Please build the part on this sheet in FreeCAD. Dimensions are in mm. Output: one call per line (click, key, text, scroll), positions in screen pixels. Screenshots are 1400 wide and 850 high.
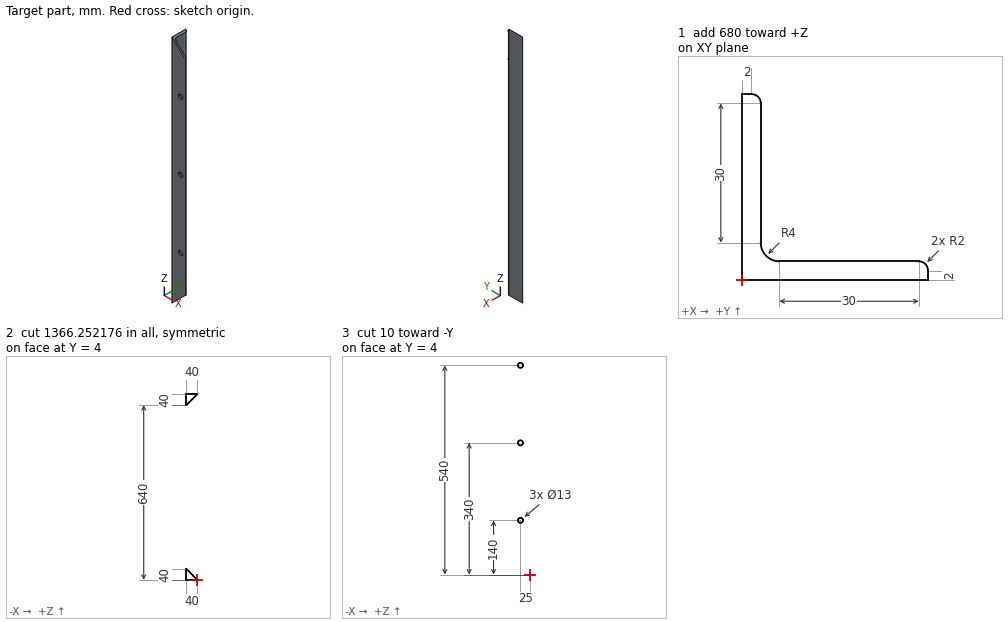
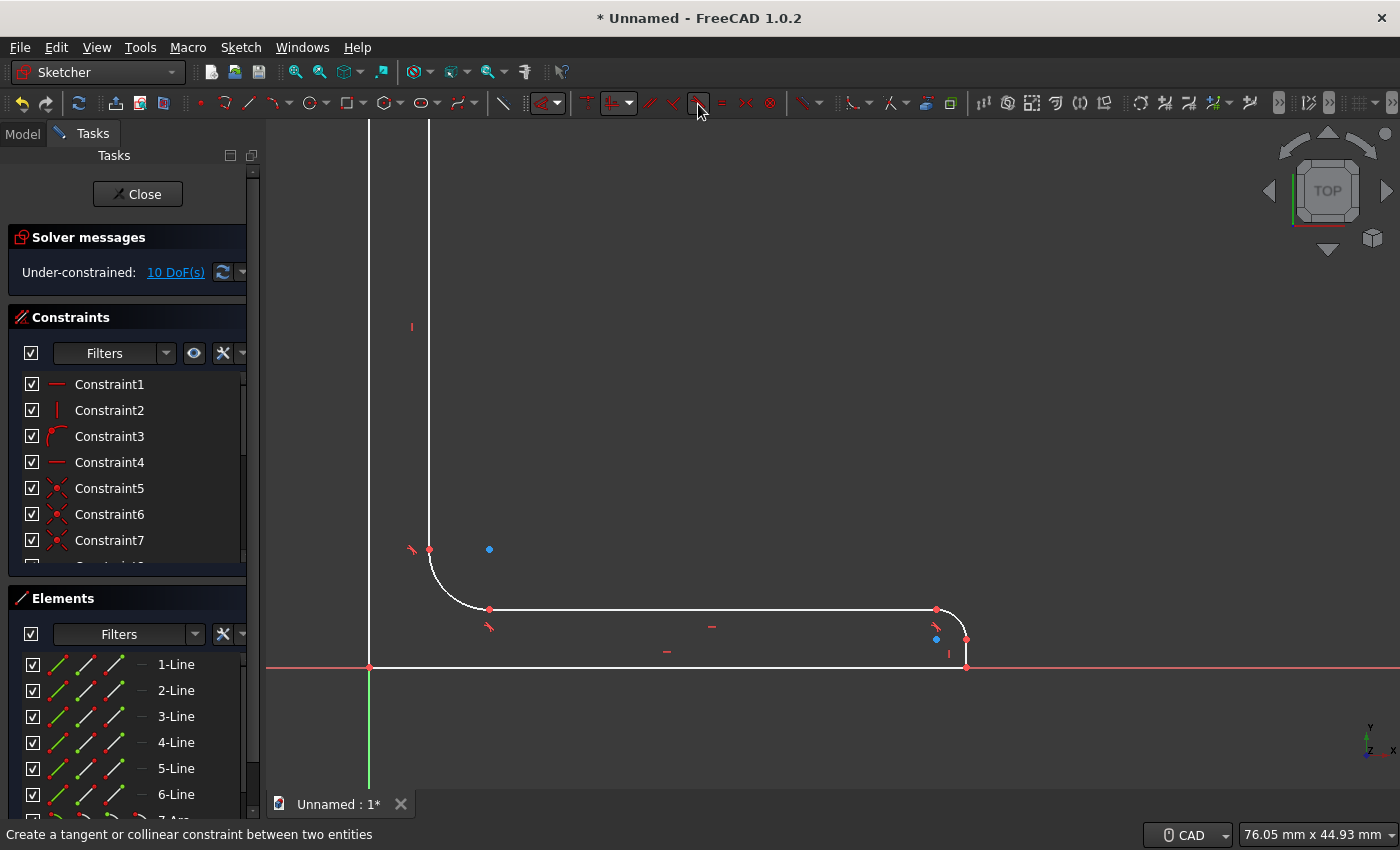
click(429, 416)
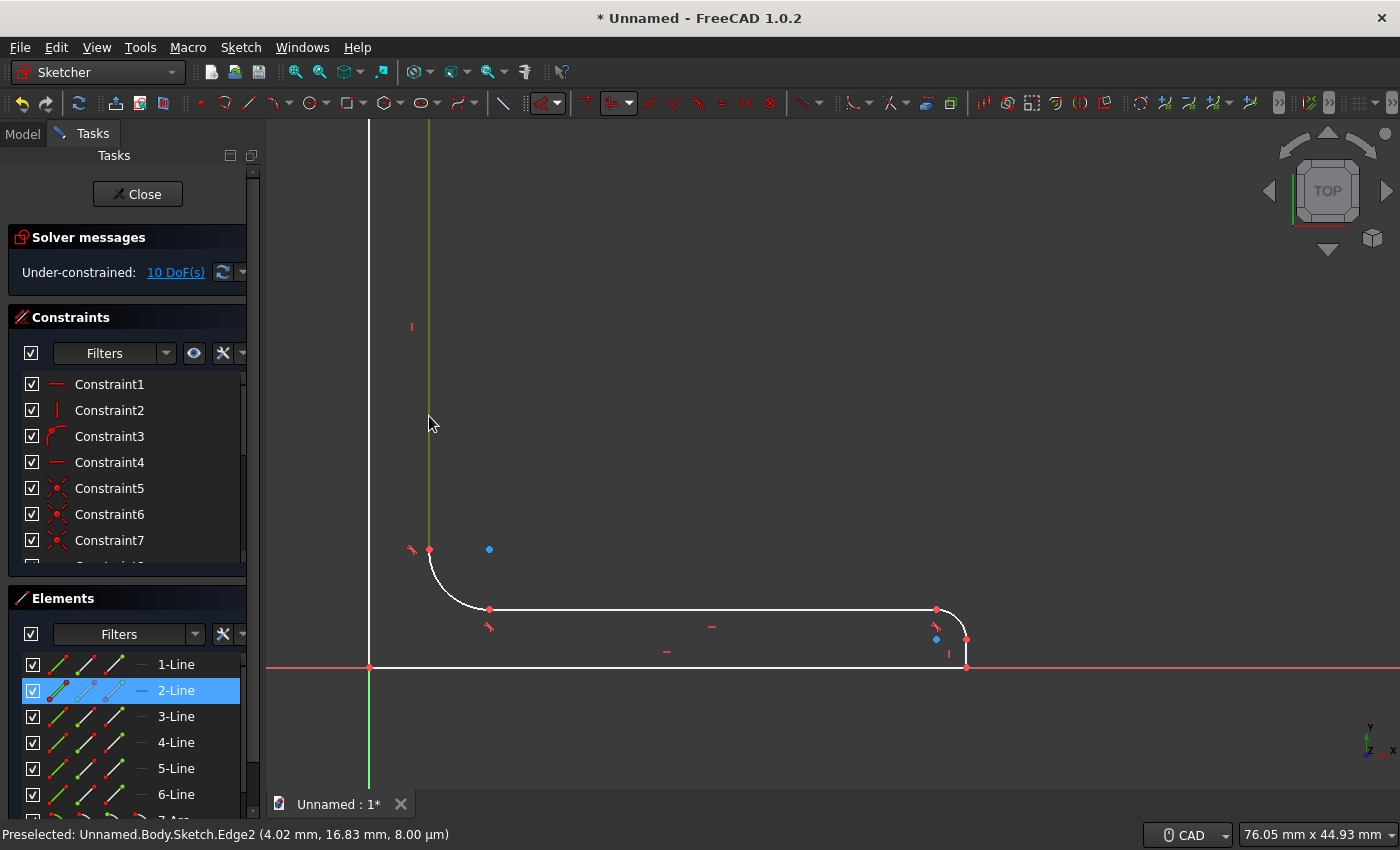
scroll(962, 625, down, 2)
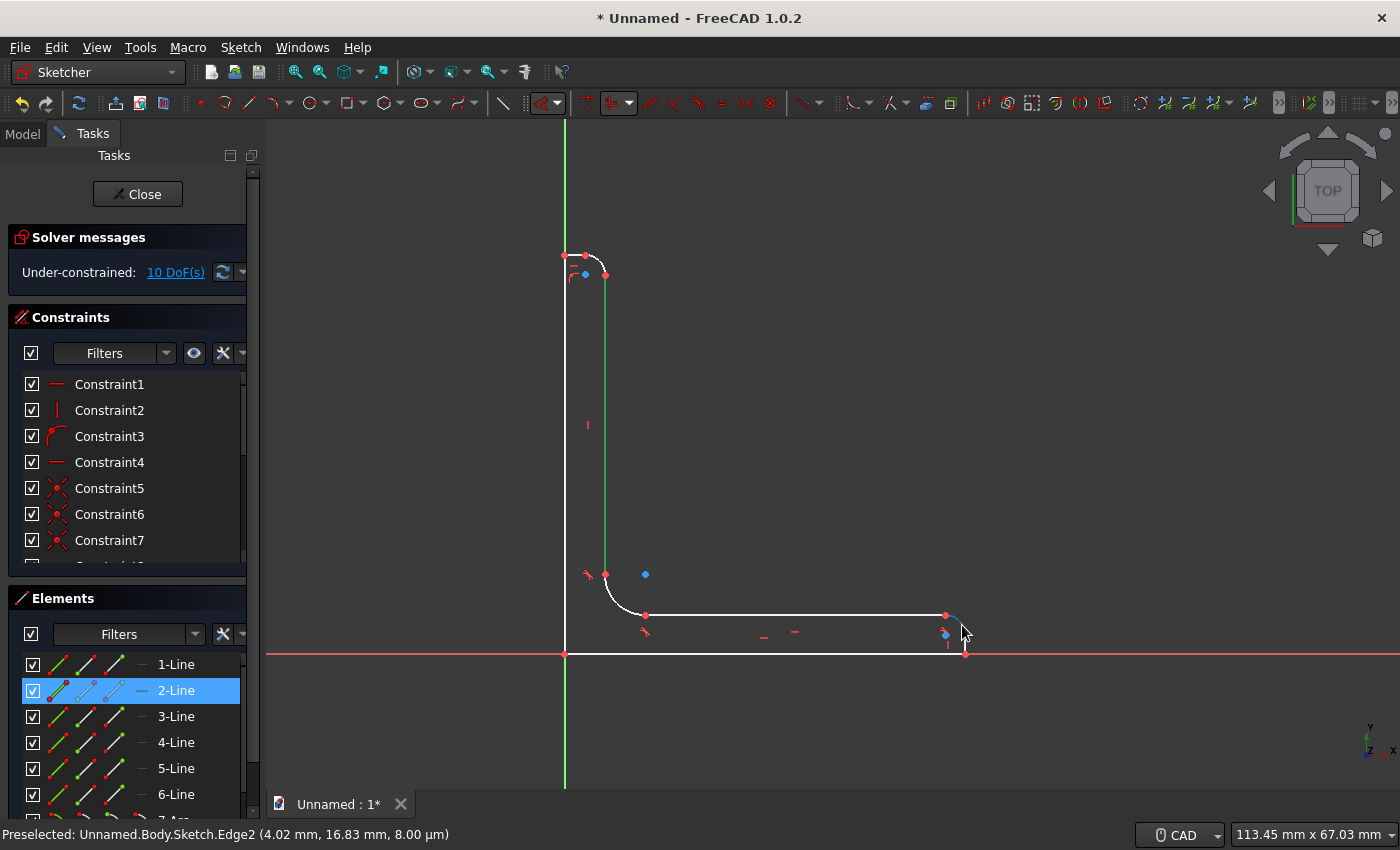
scroll(603, 266, up, 2)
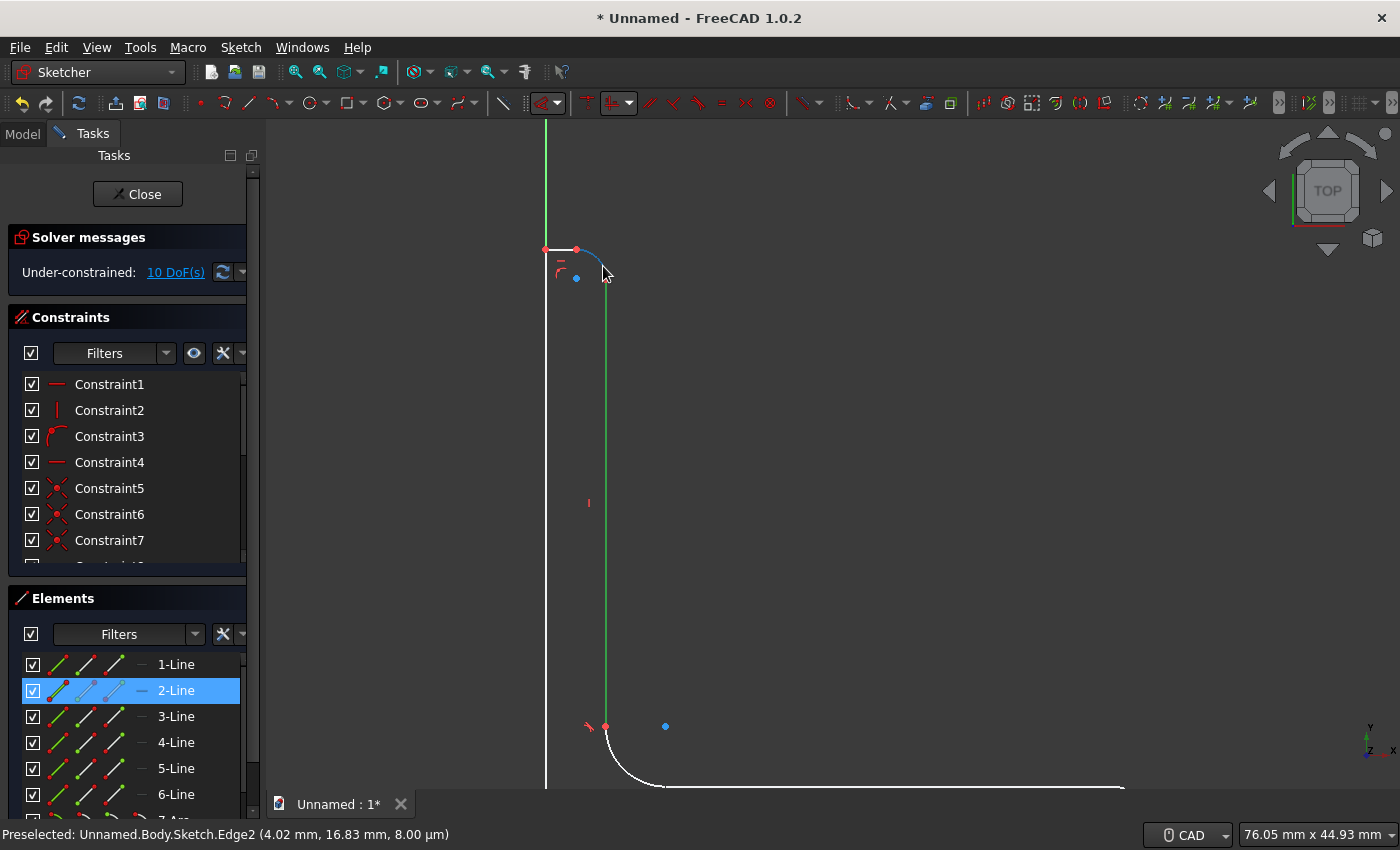
click(603, 266)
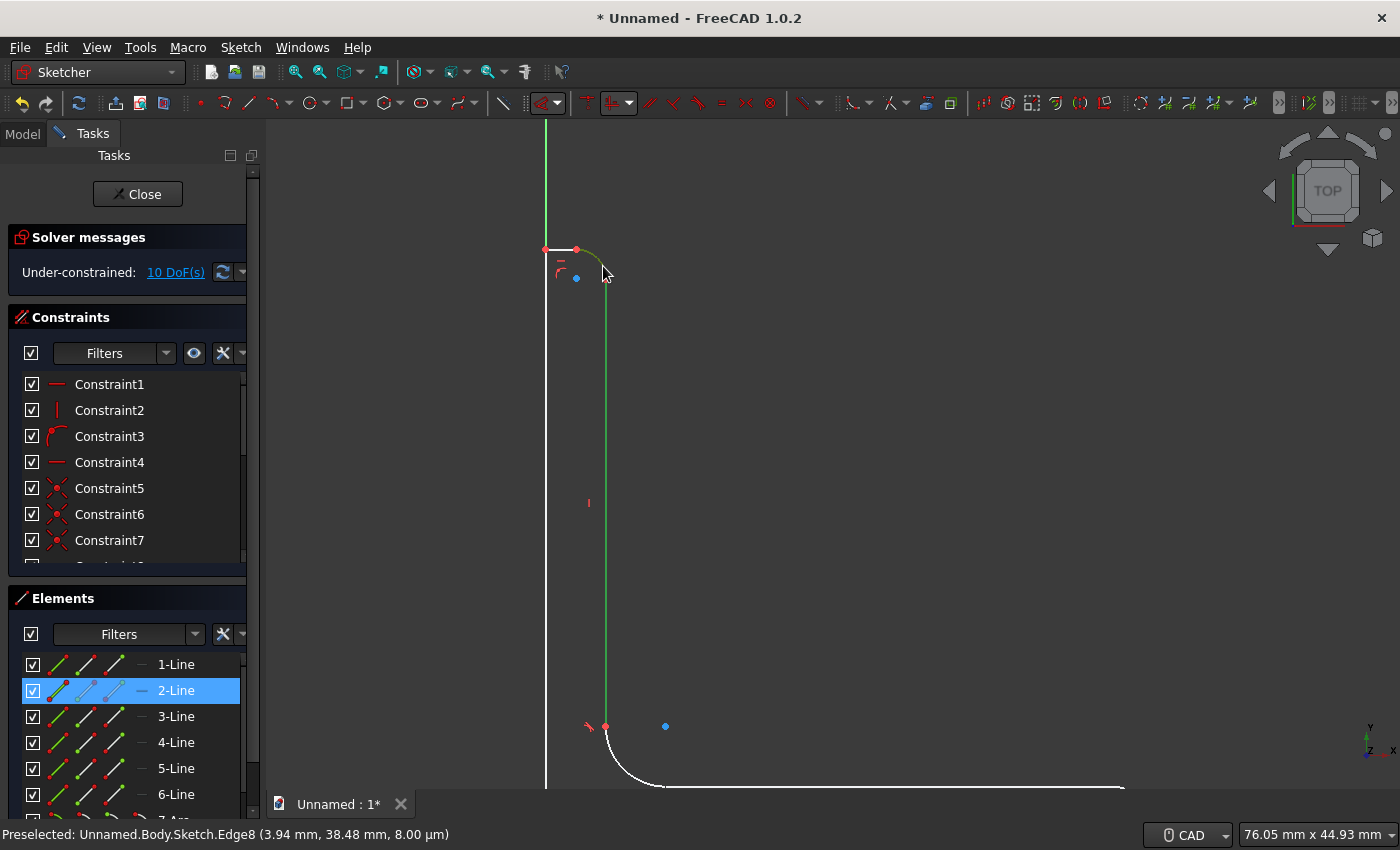
click(698, 104)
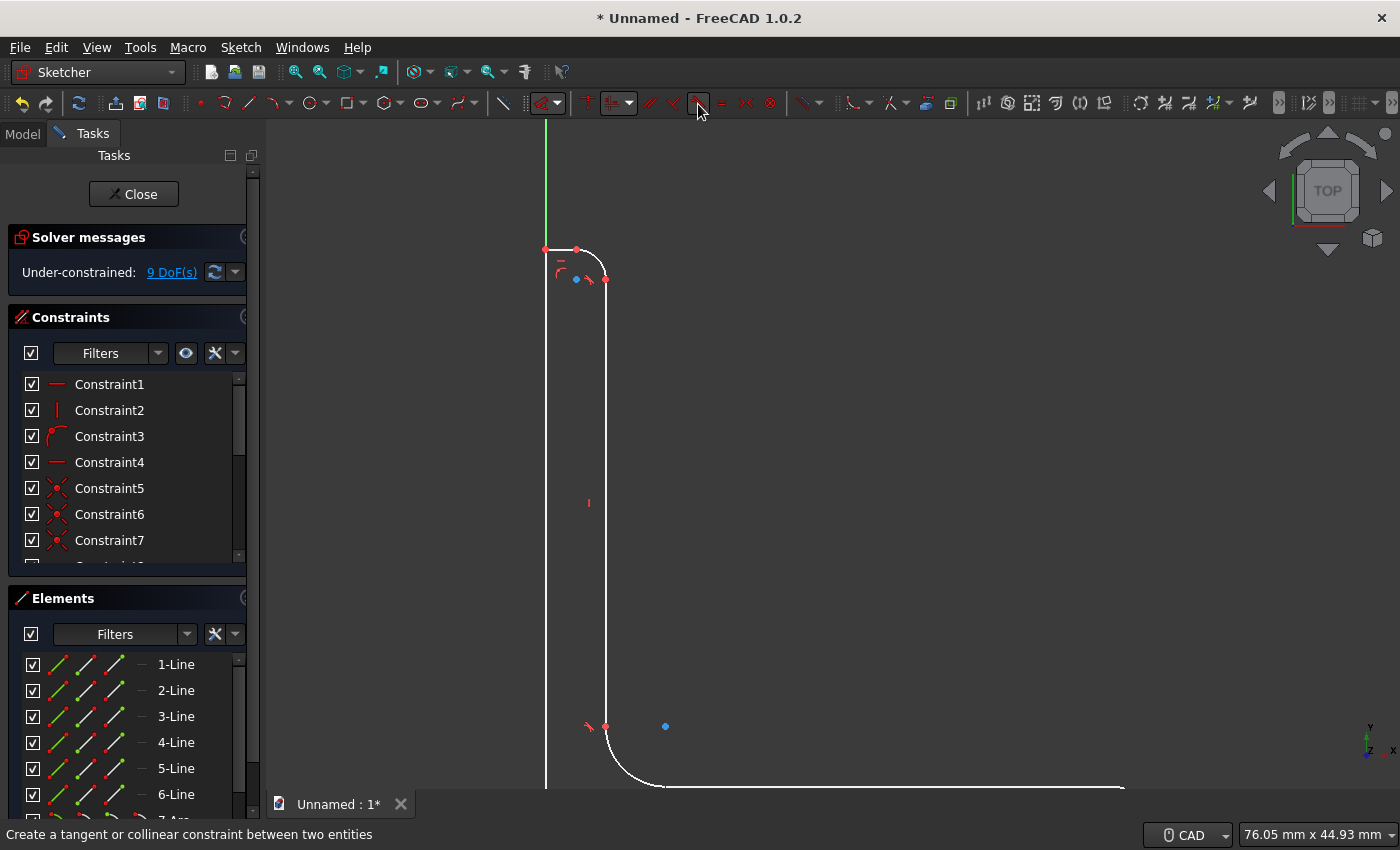
scroll(567, 250, up, 3)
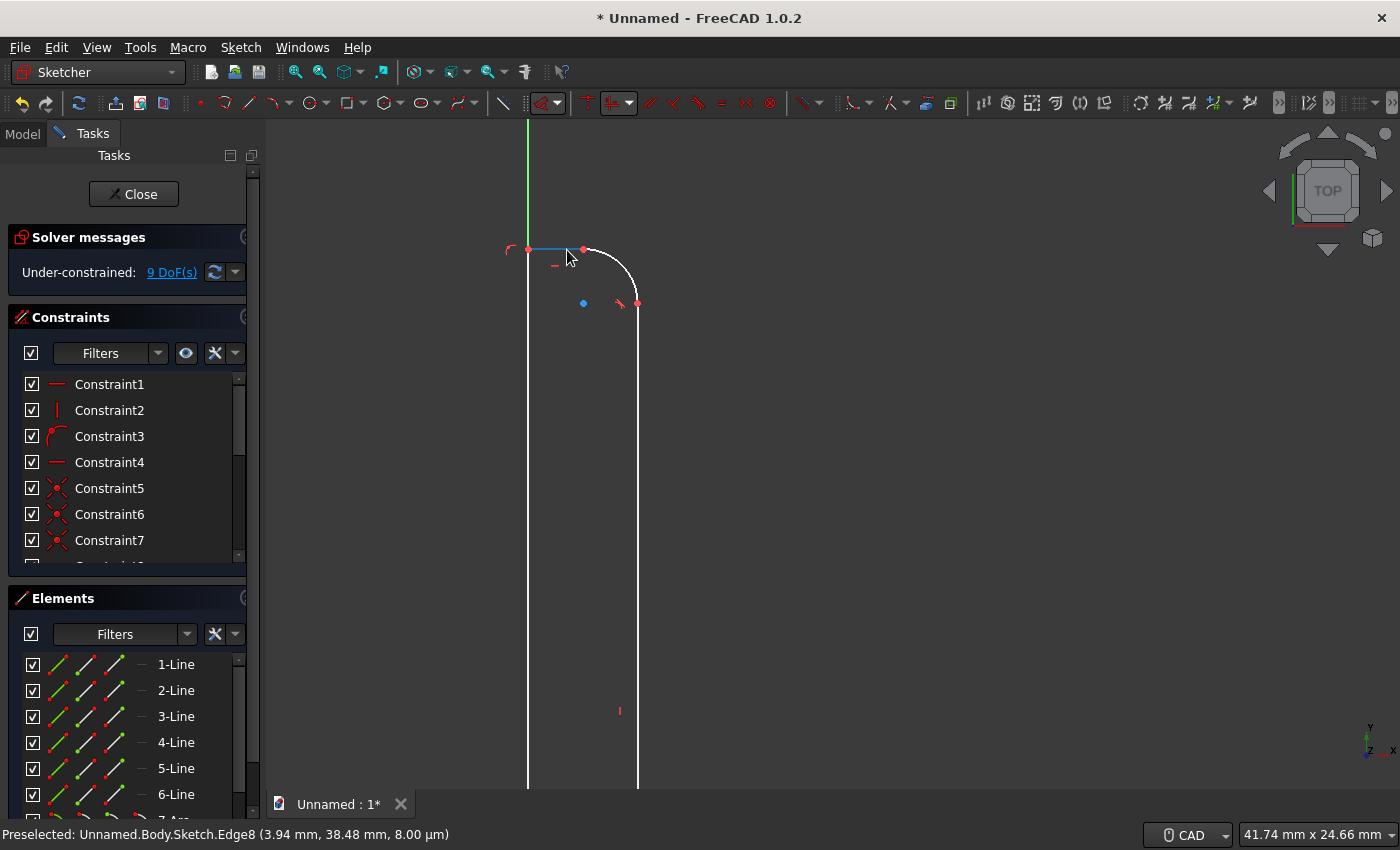
click(567, 249)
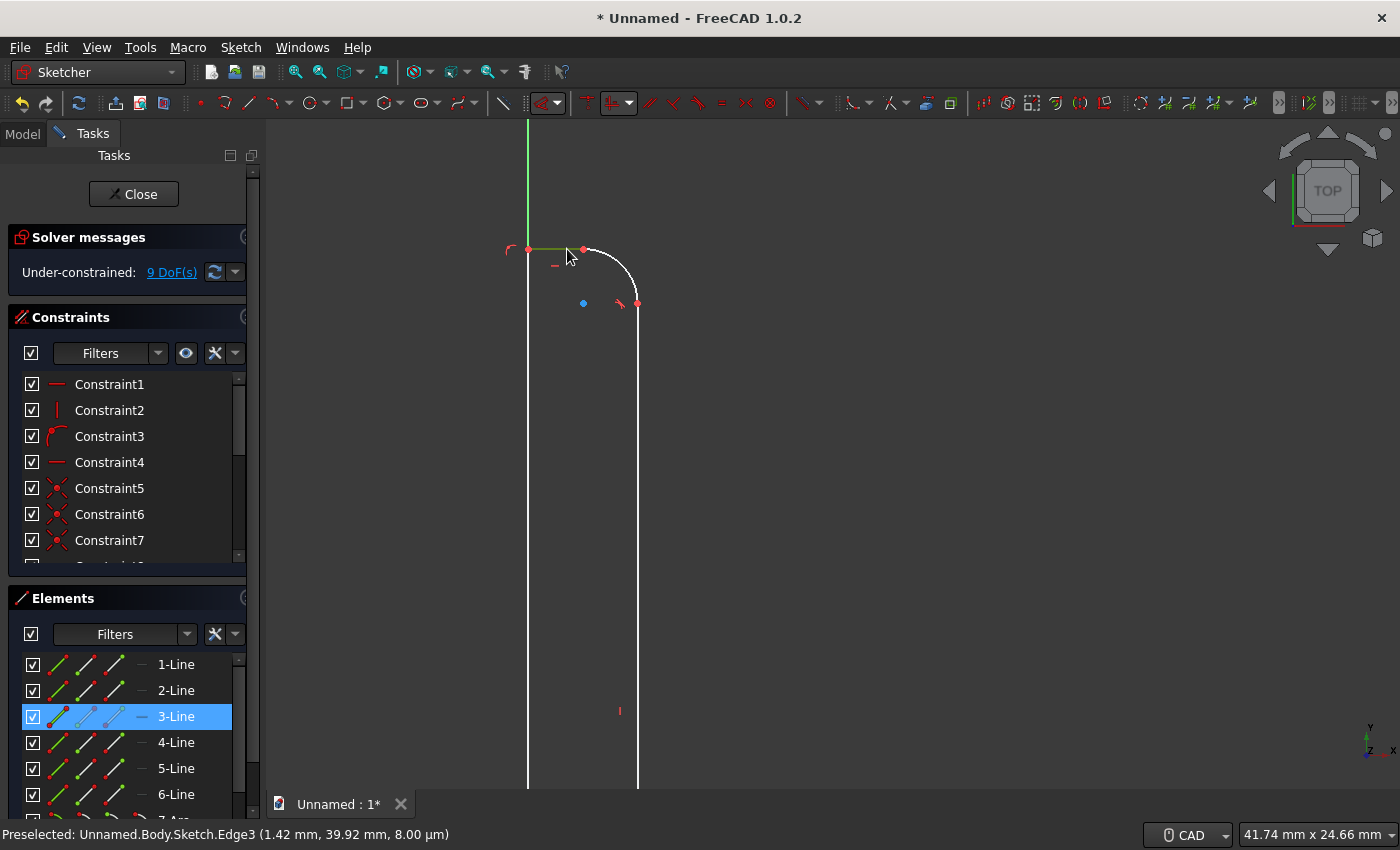
click(632, 279)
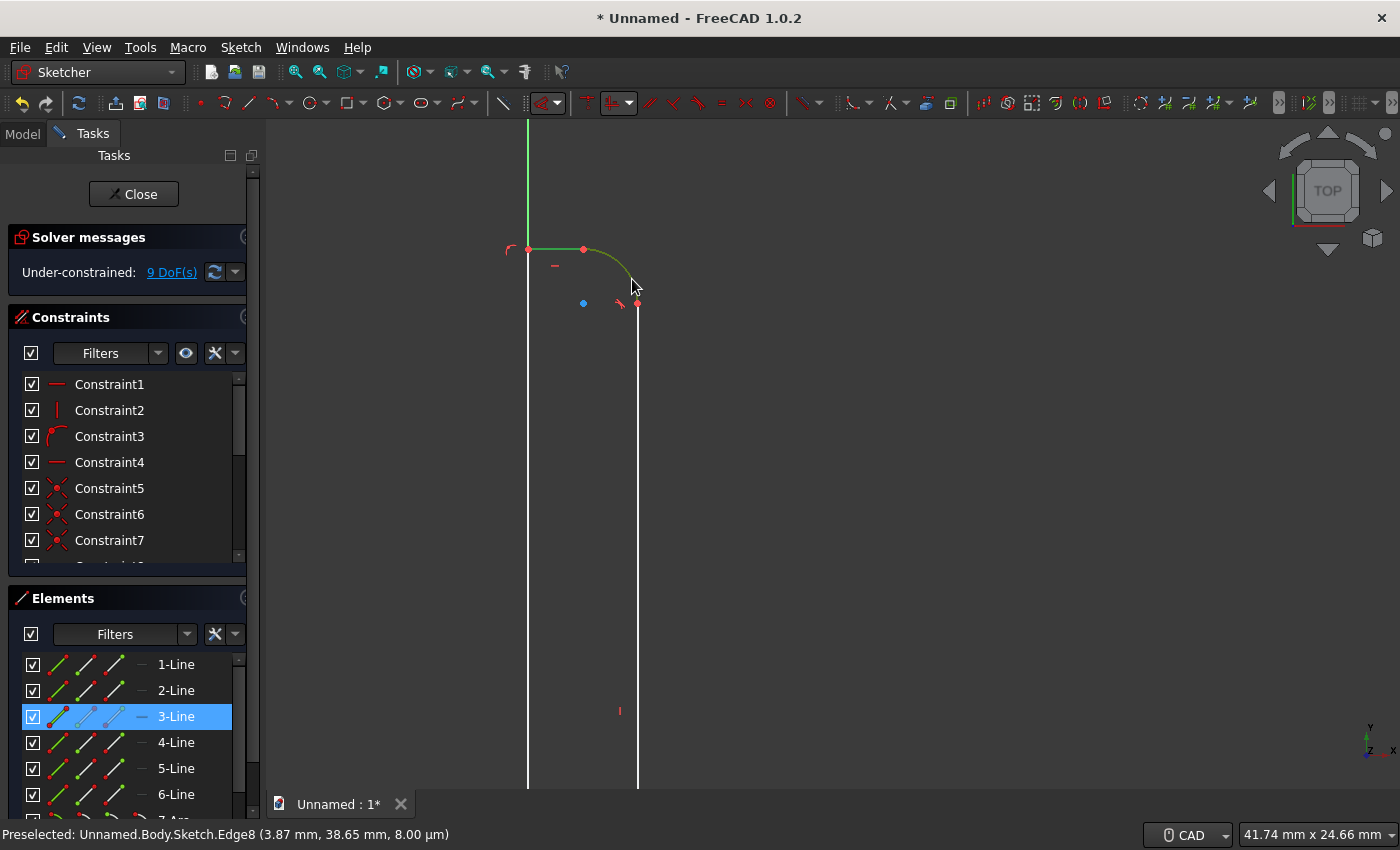
click(698, 104)